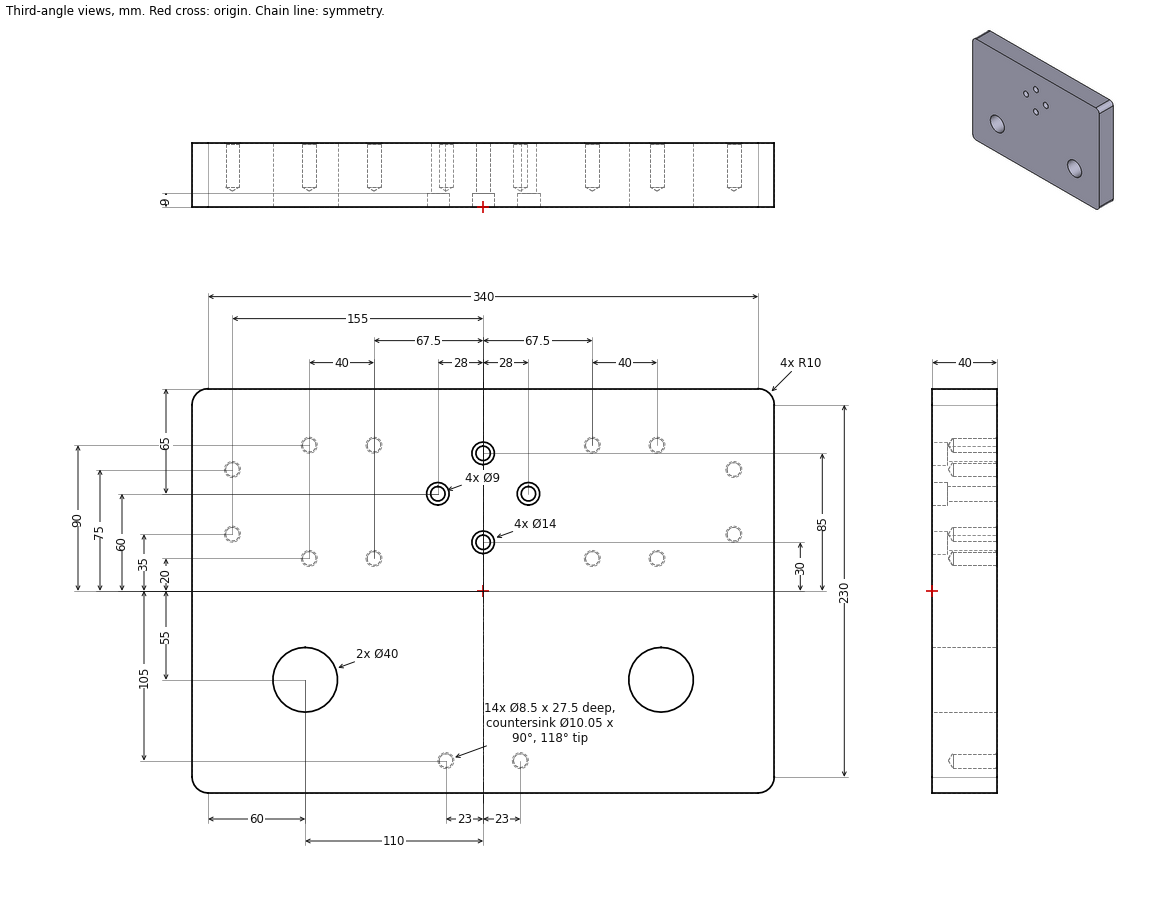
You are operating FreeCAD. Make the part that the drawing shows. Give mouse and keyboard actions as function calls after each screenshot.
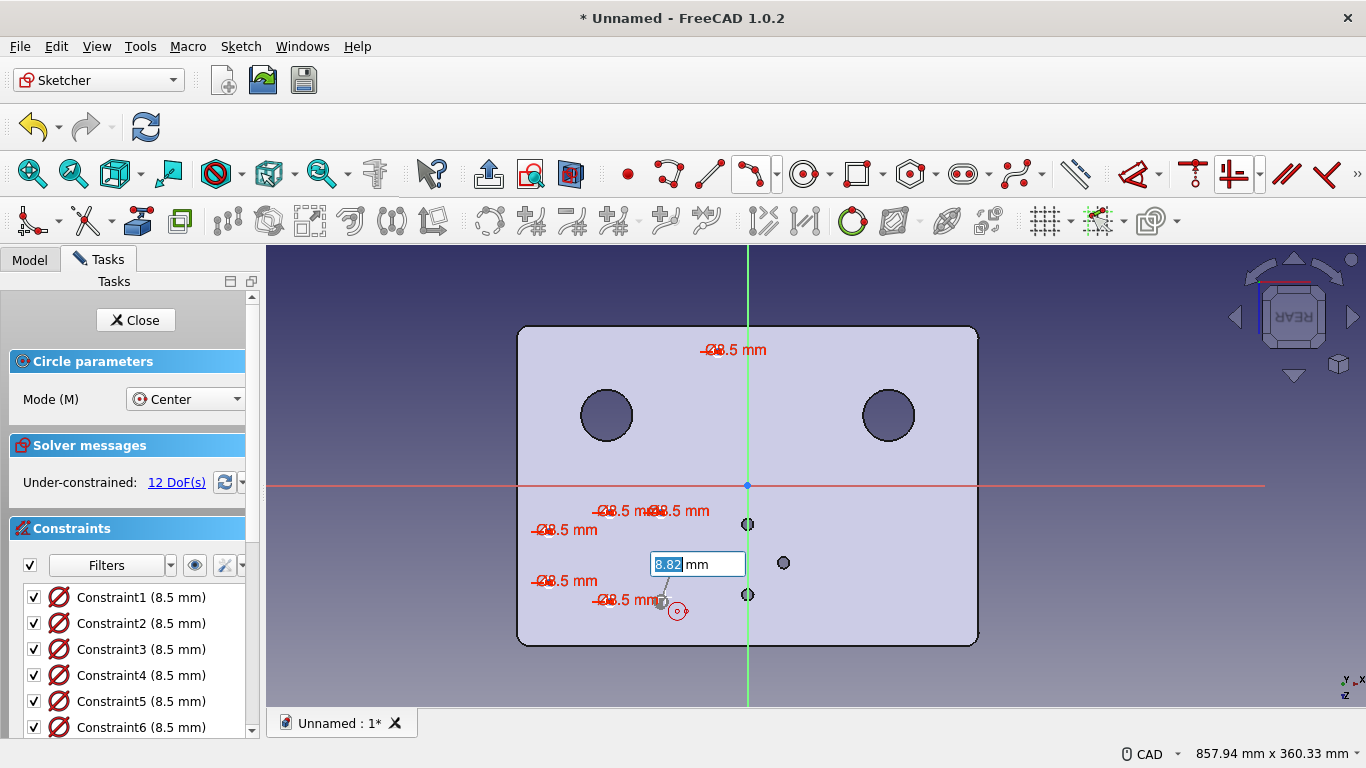
text(8.5)
key(Return)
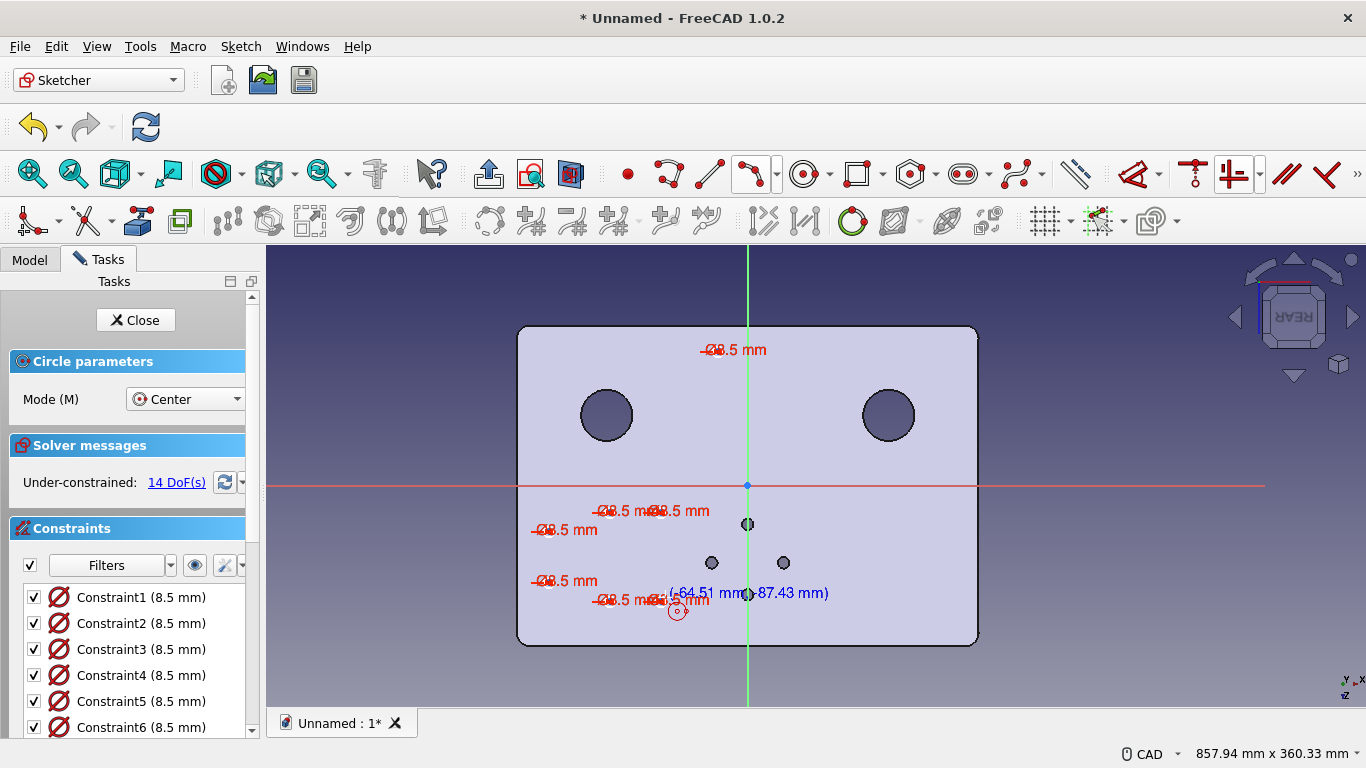
scroll(946, 582, up, 8)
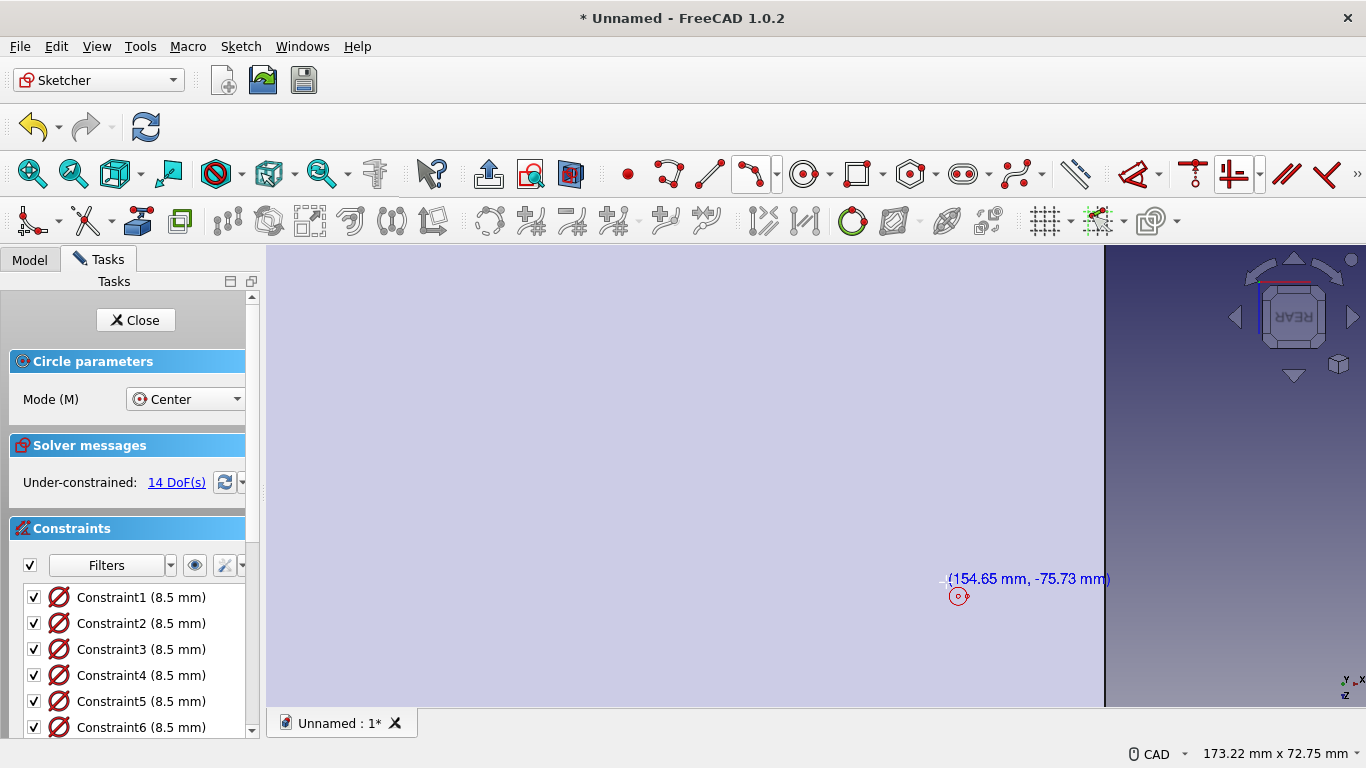
scroll(946, 582, down, 8)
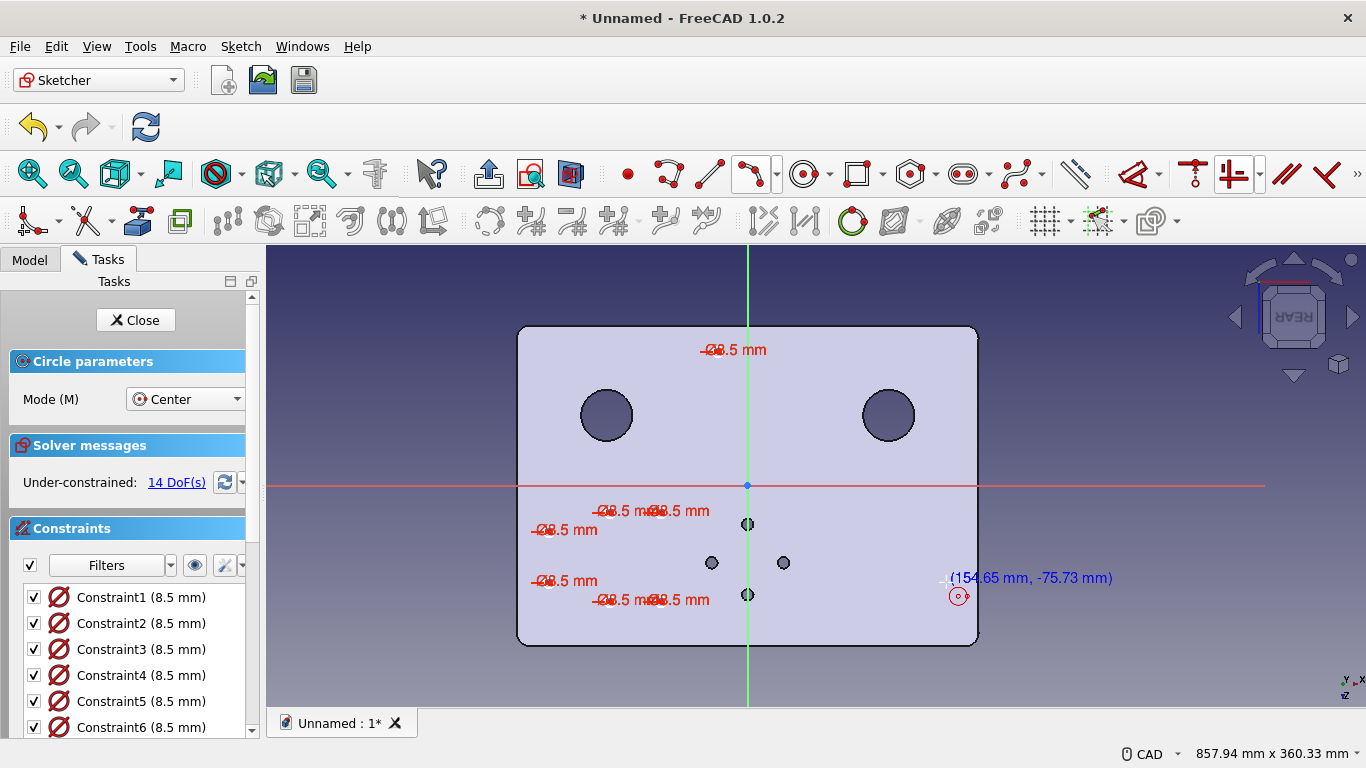
click(946, 582)
move(950, 578)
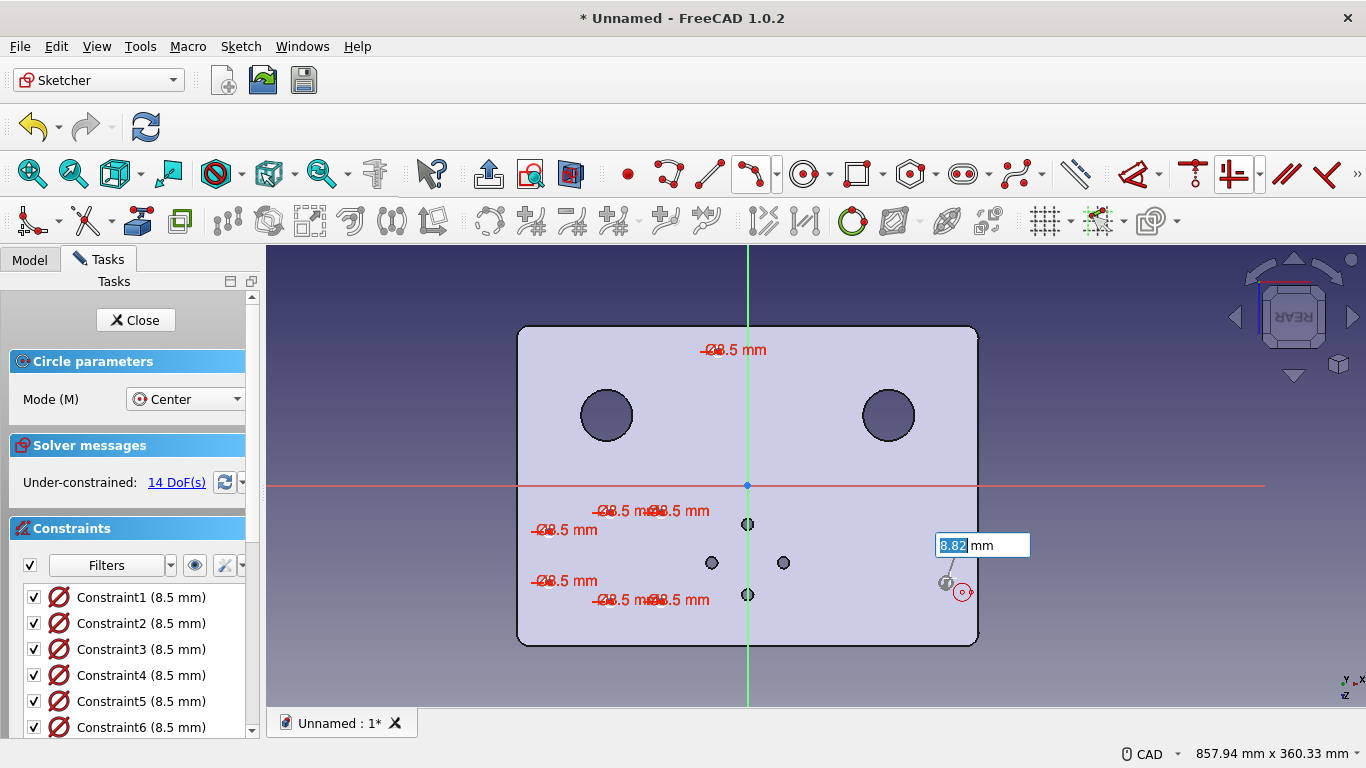
text(8.5)
key(Return)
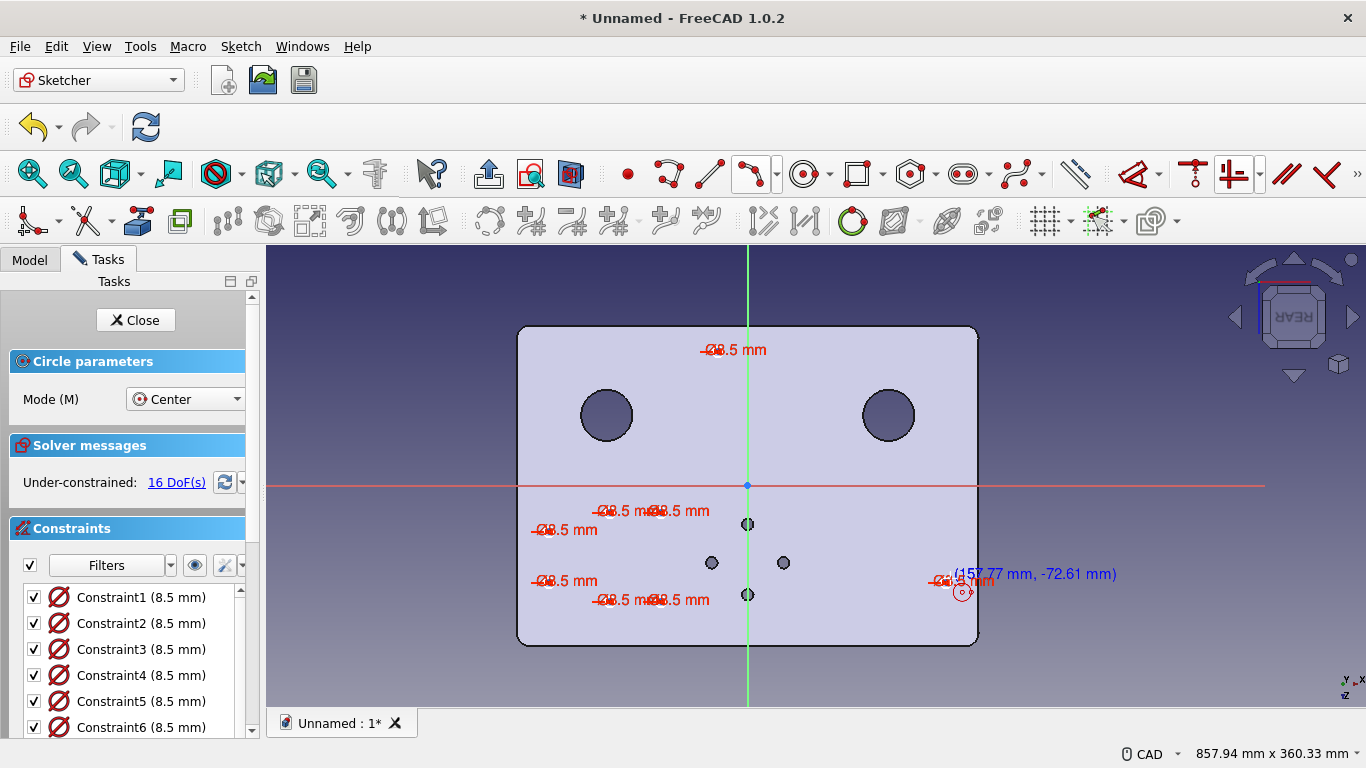
scroll(946, 531, up, 8)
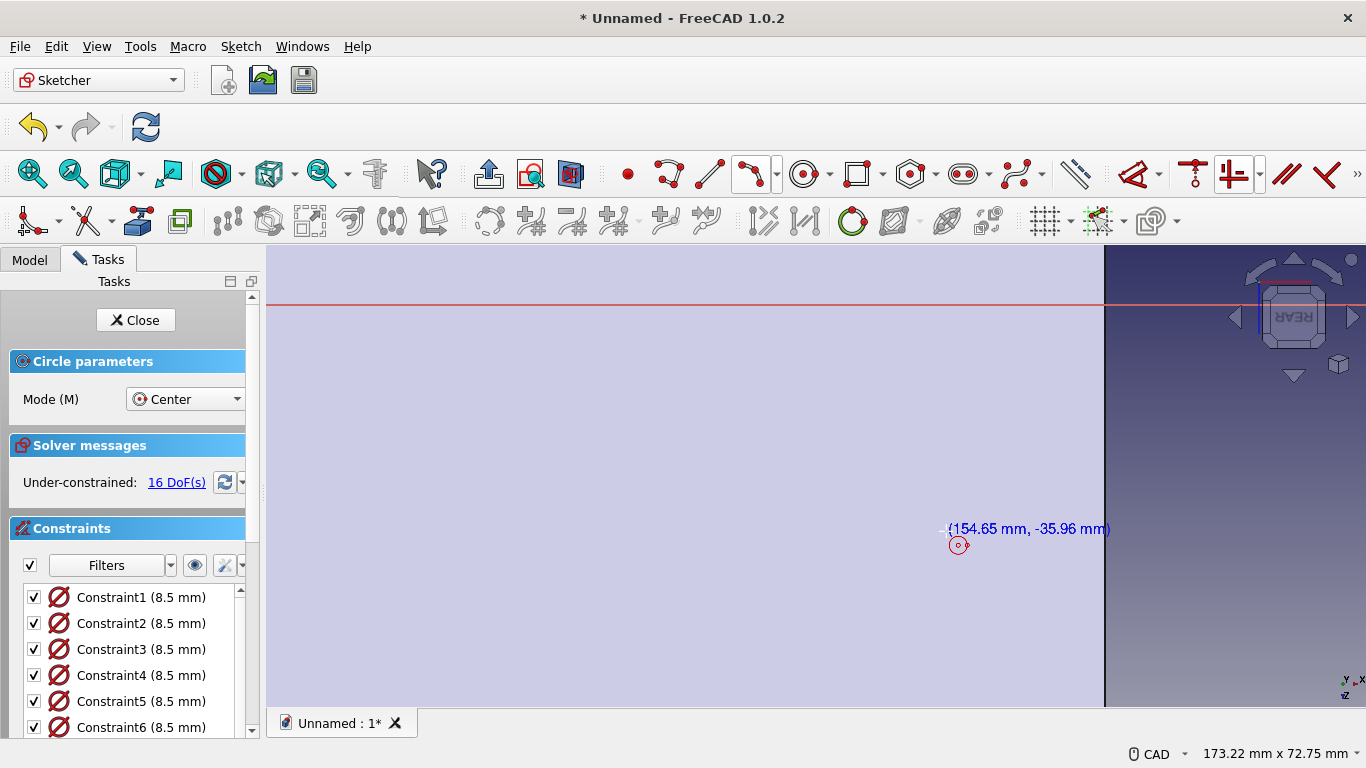
scroll(946, 531, down, 8)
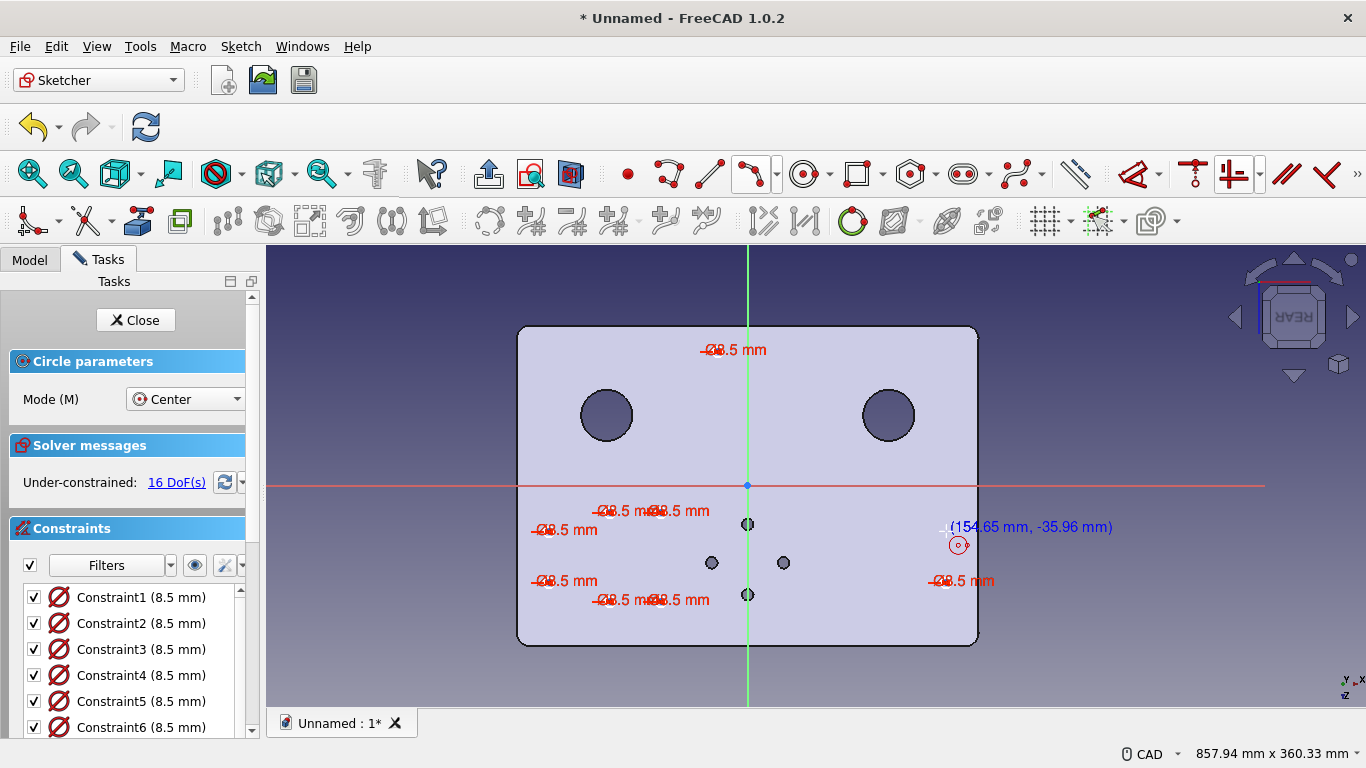
click(946, 531)
move(950, 527)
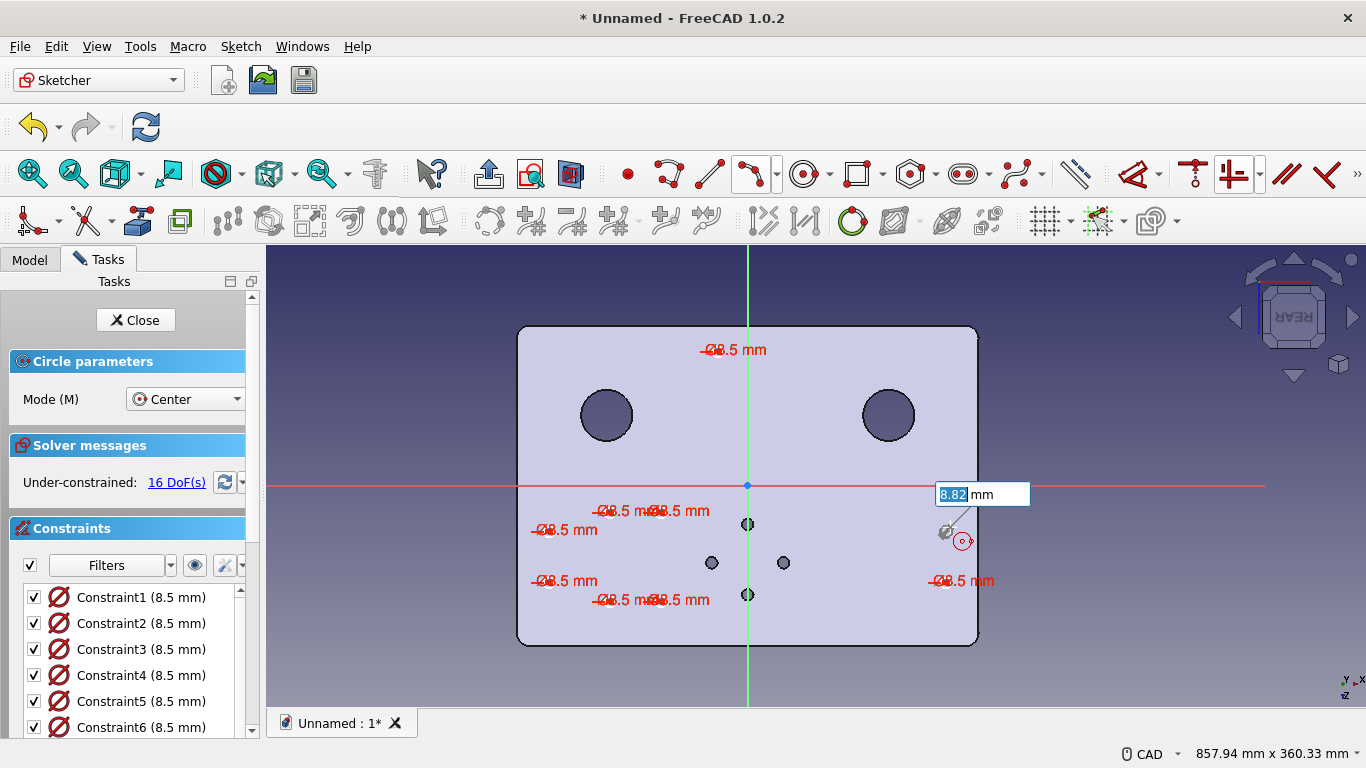
text(8.5)
key(Return)